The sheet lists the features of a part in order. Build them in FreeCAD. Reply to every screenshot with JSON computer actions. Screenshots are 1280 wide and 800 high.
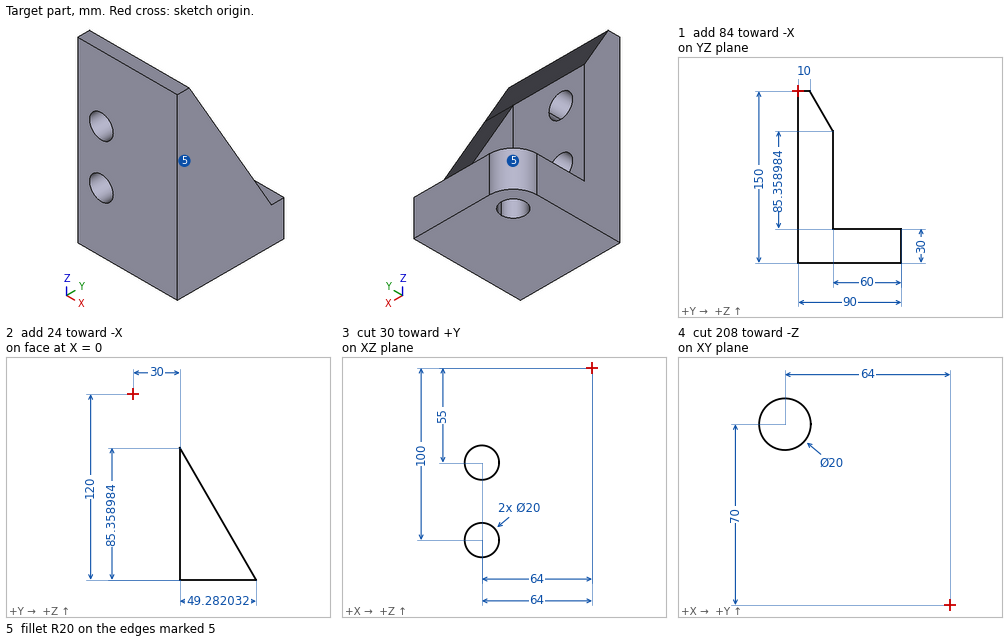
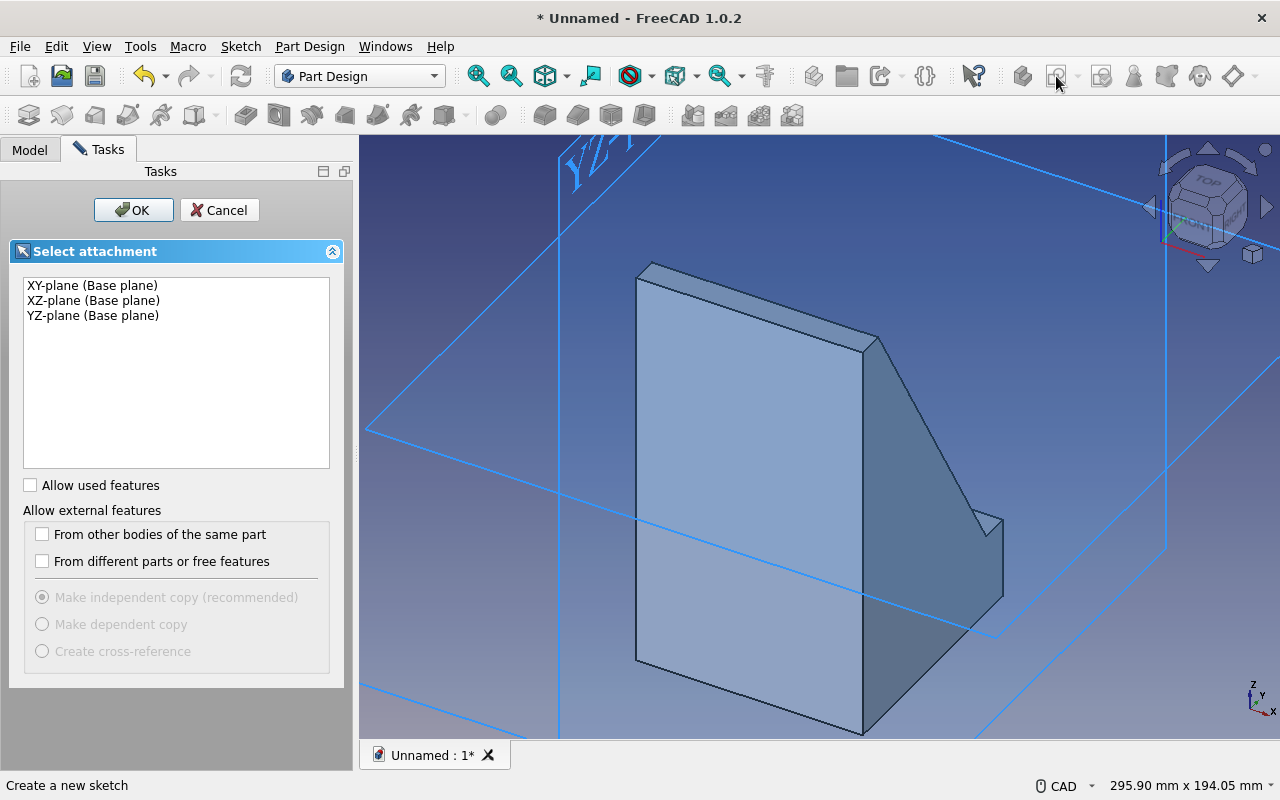
{"action": "left_click", "coordinate": [84, 300]}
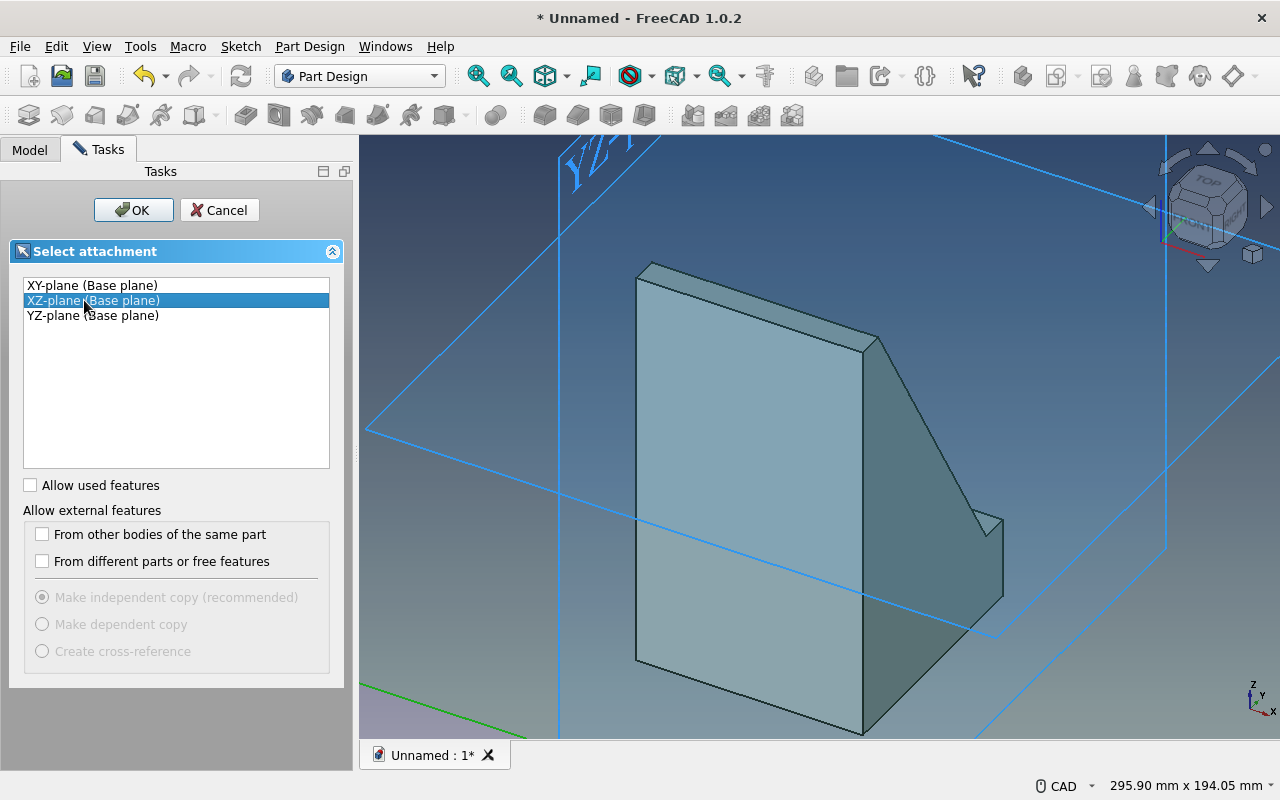
{"action": "left_click", "coordinate": [134, 210]}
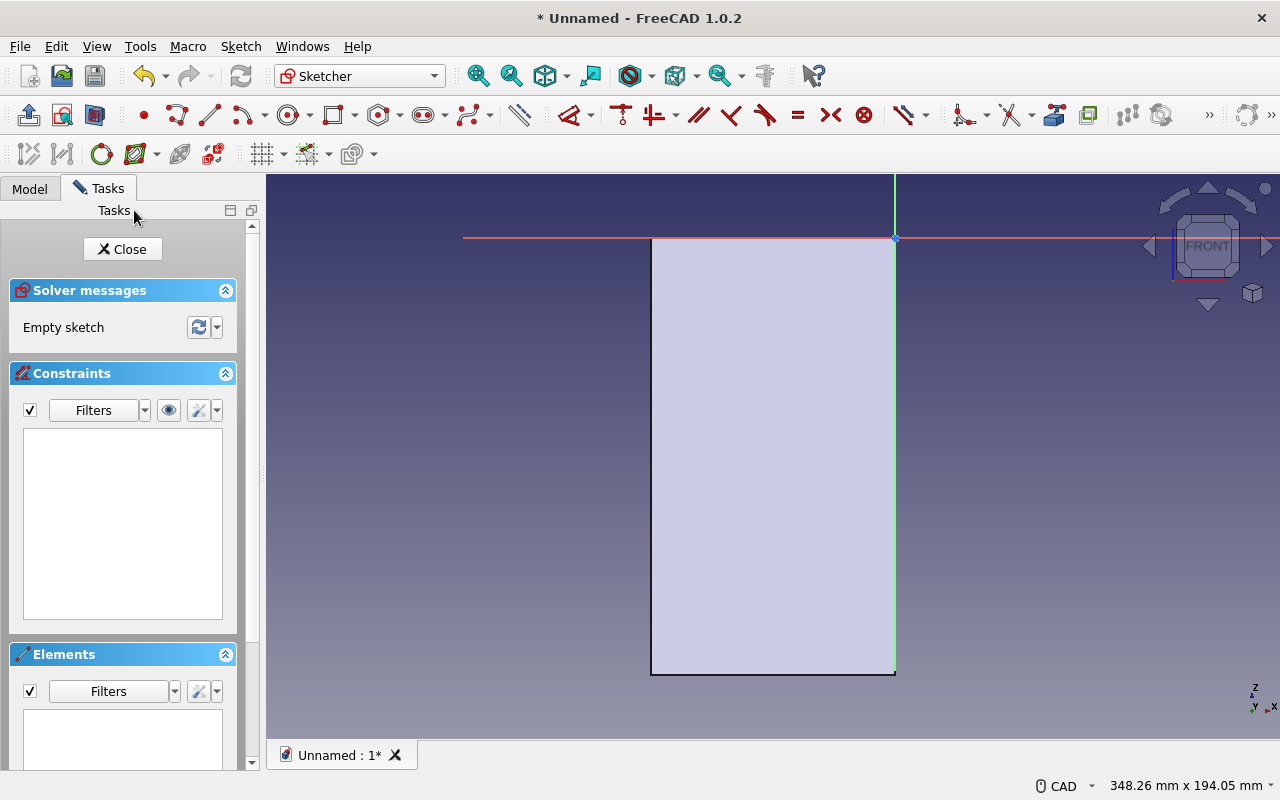
{"action": "left_click", "coordinate": [288, 116]}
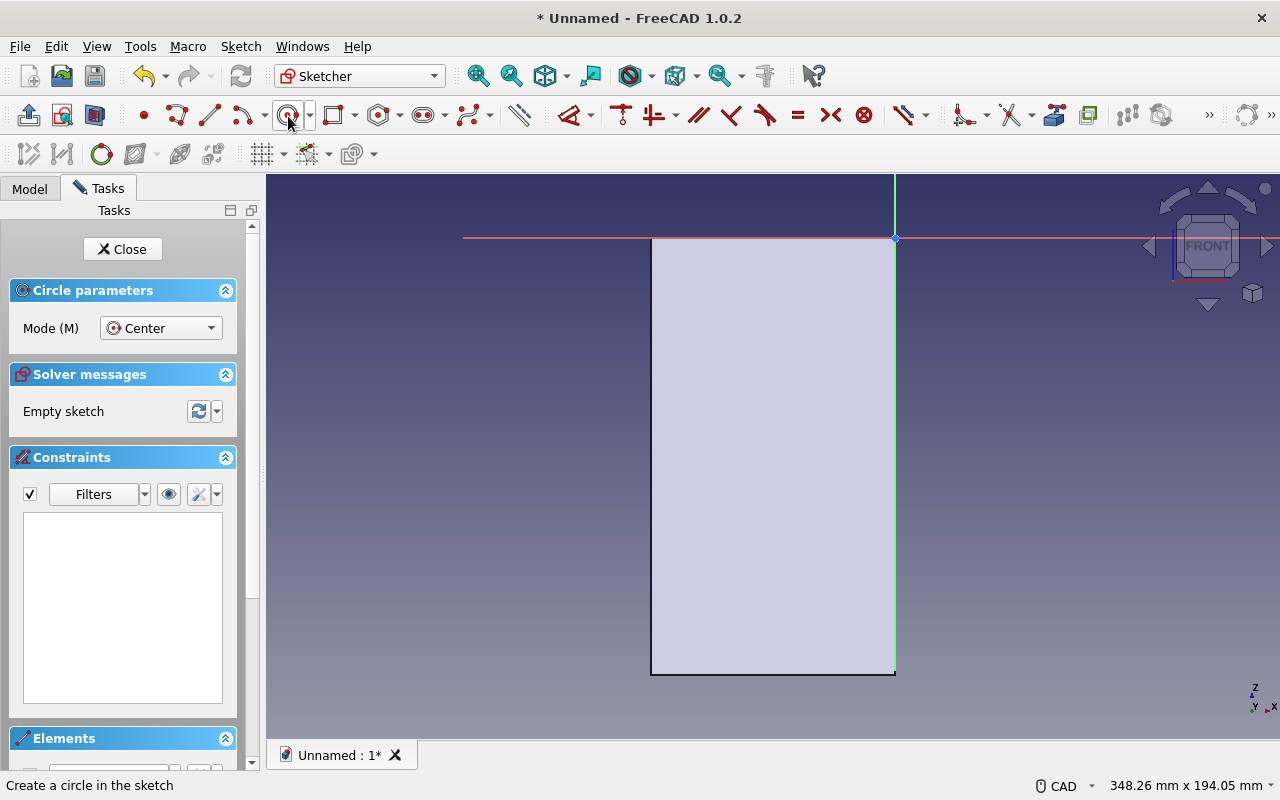
{"action": "left_click", "coordinate": [709, 529]}
{"action": "left_click", "coordinate": [730, 509]}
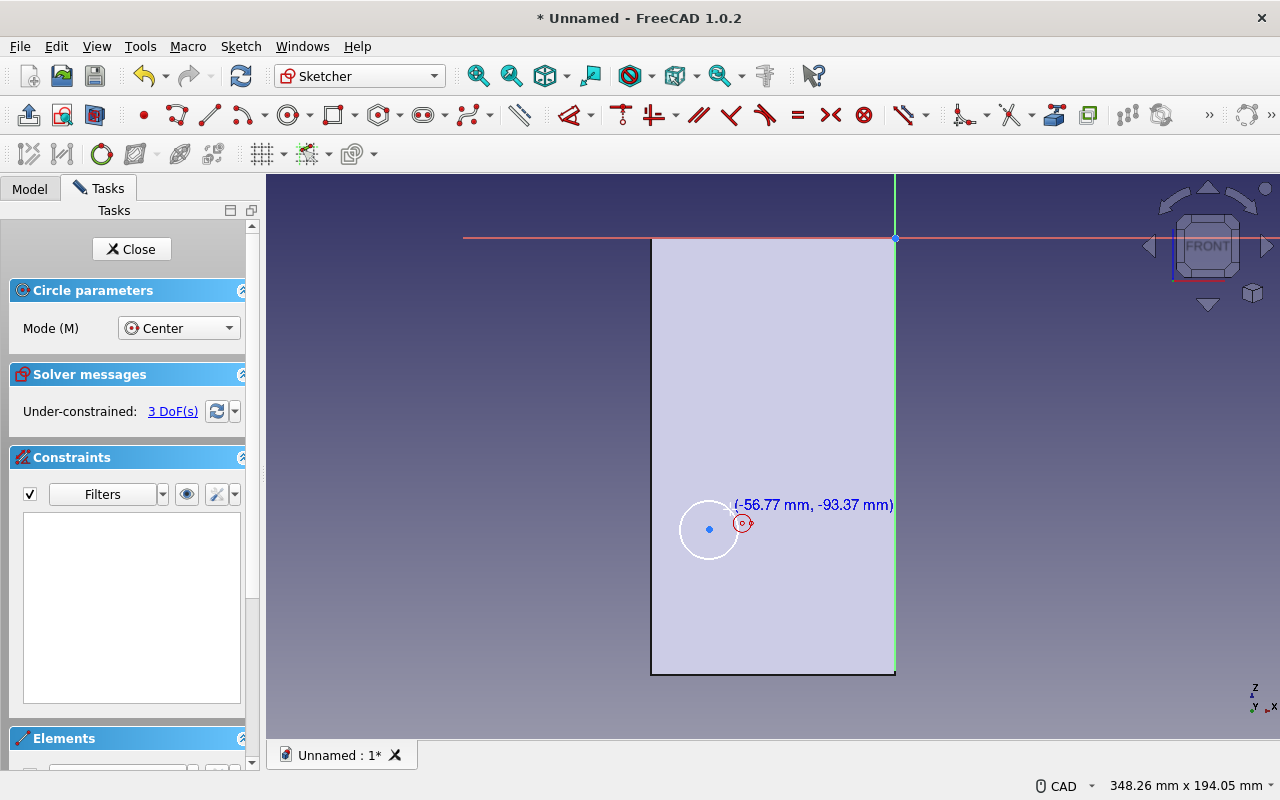
{"action": "left_click", "coordinate": [709, 398]}
{"action": "left_click", "coordinate": [730, 378]}
{"action": "key", "text": "Escape"}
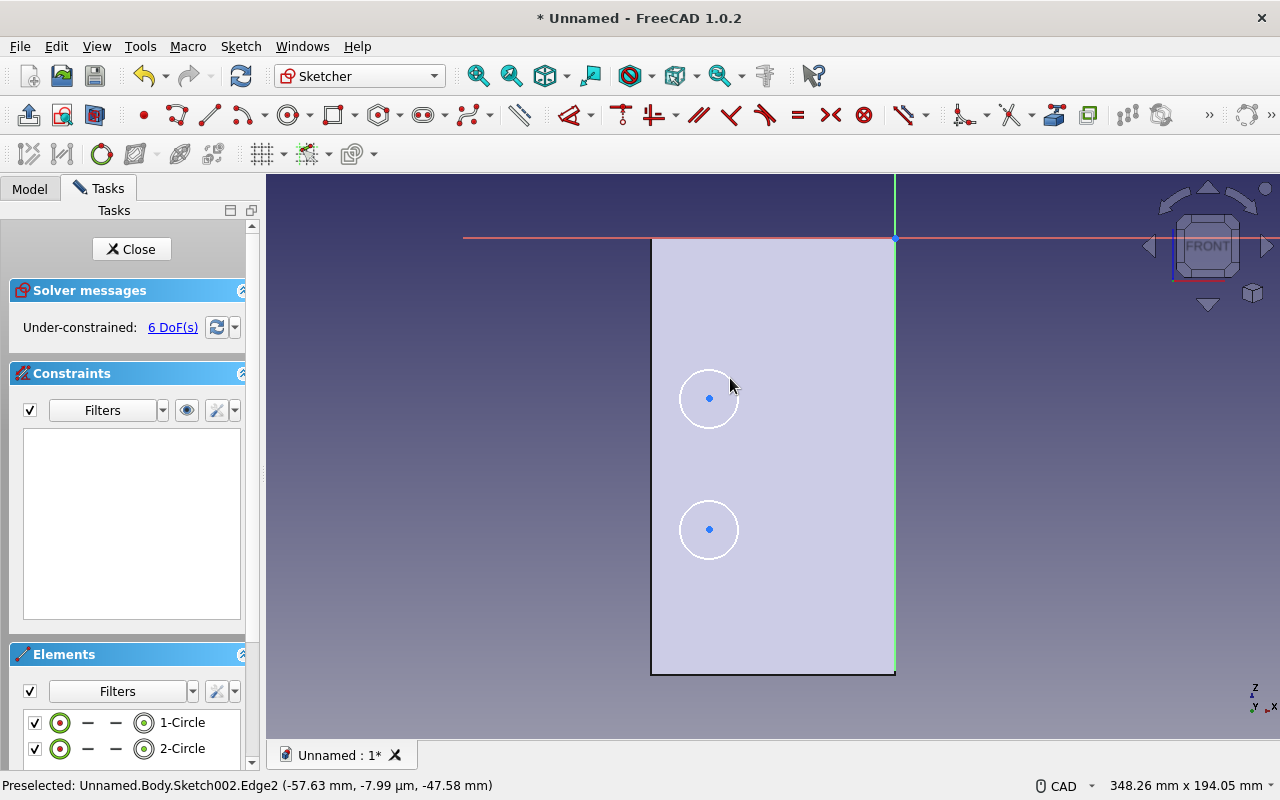
{"action": "left_click", "coordinate": [729, 509]}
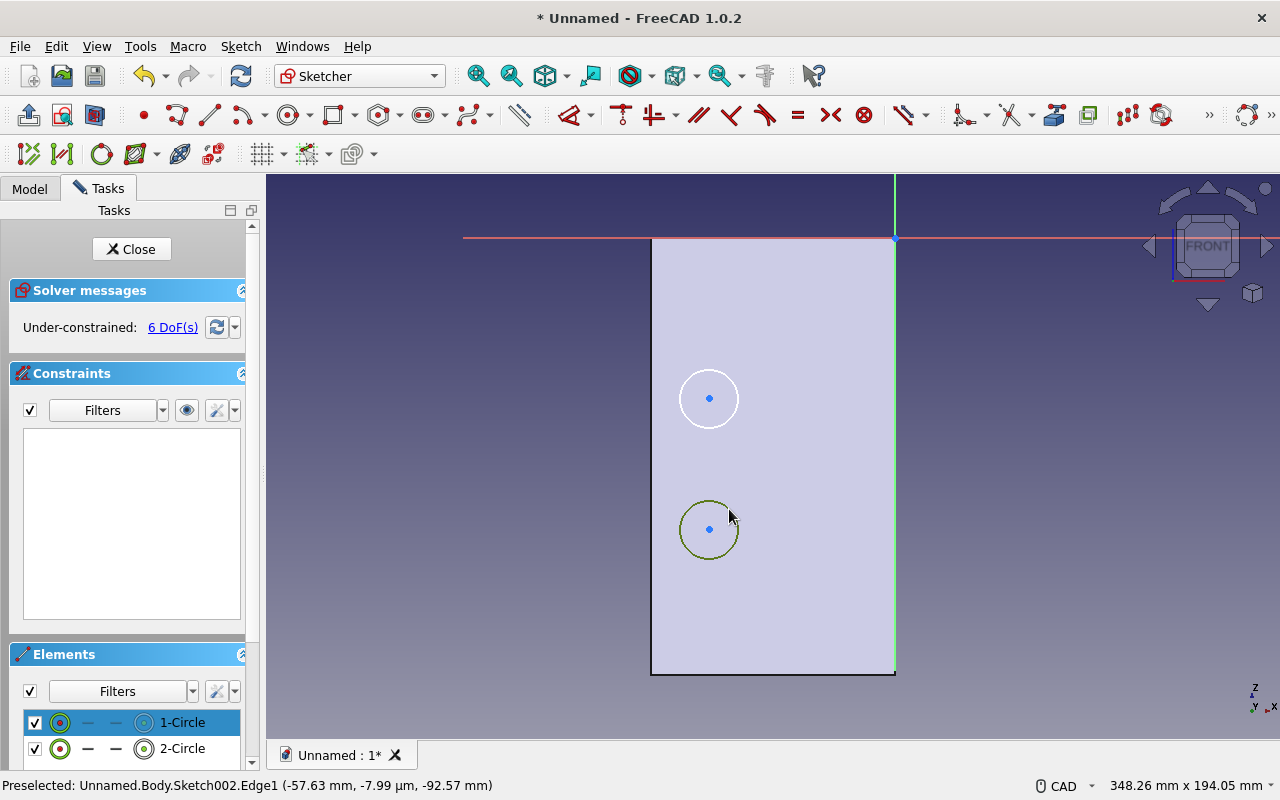
{"action": "left_click", "coordinate": [729, 378]}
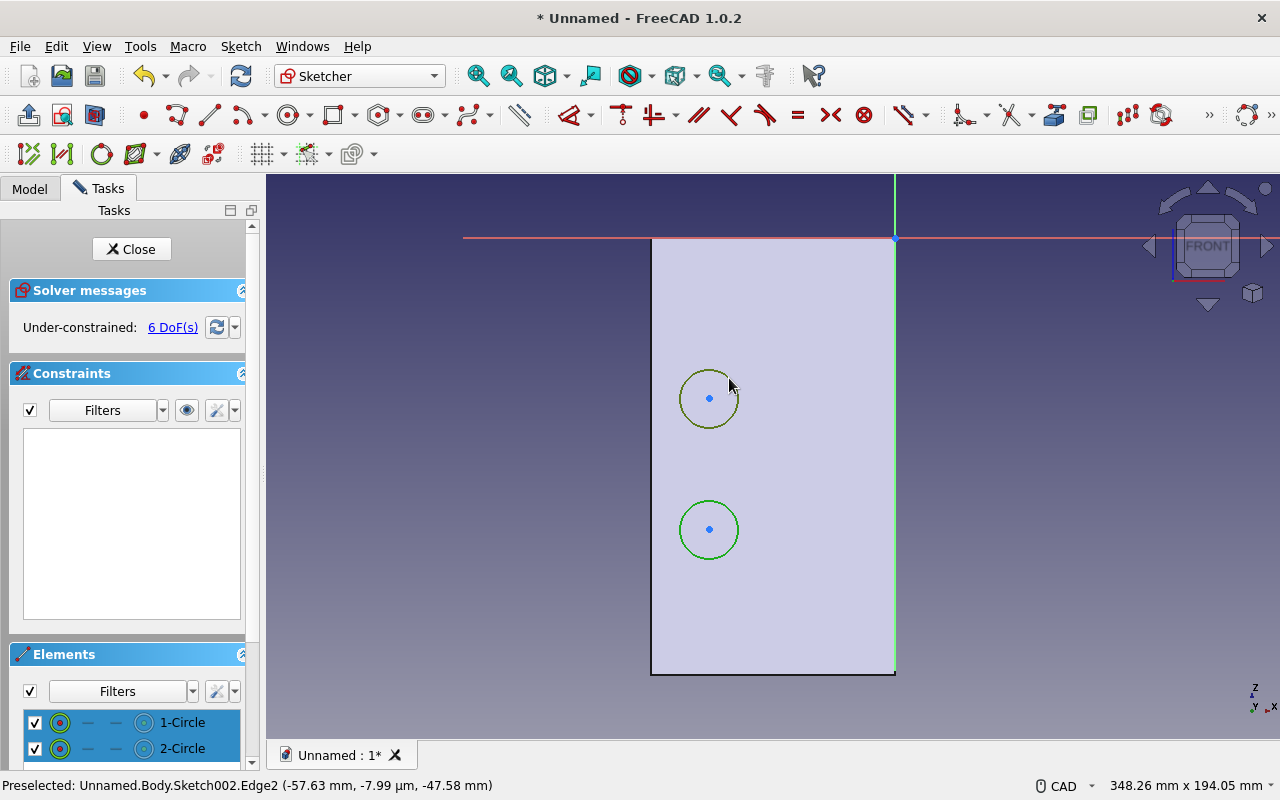
{"action": "left_click", "coordinate": [798, 116]}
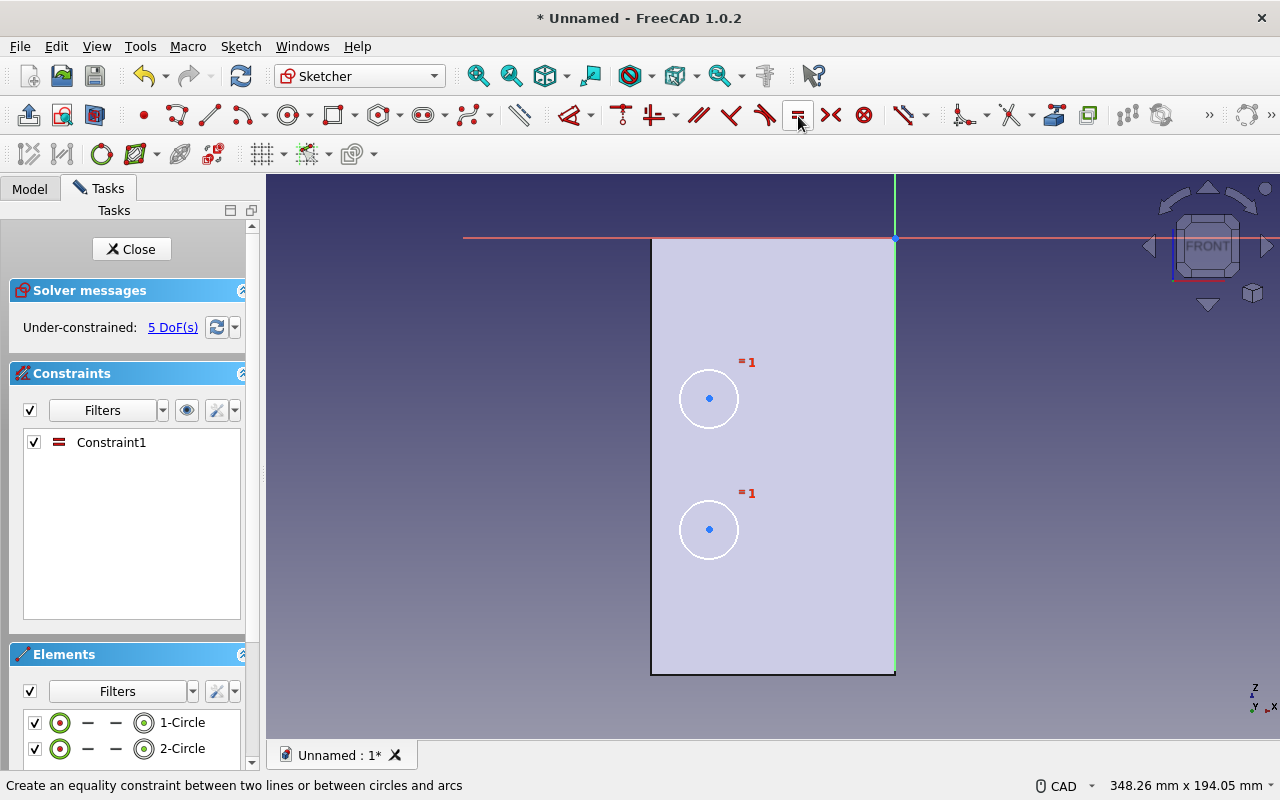
{"action": "left_click", "coordinate": [568, 116]}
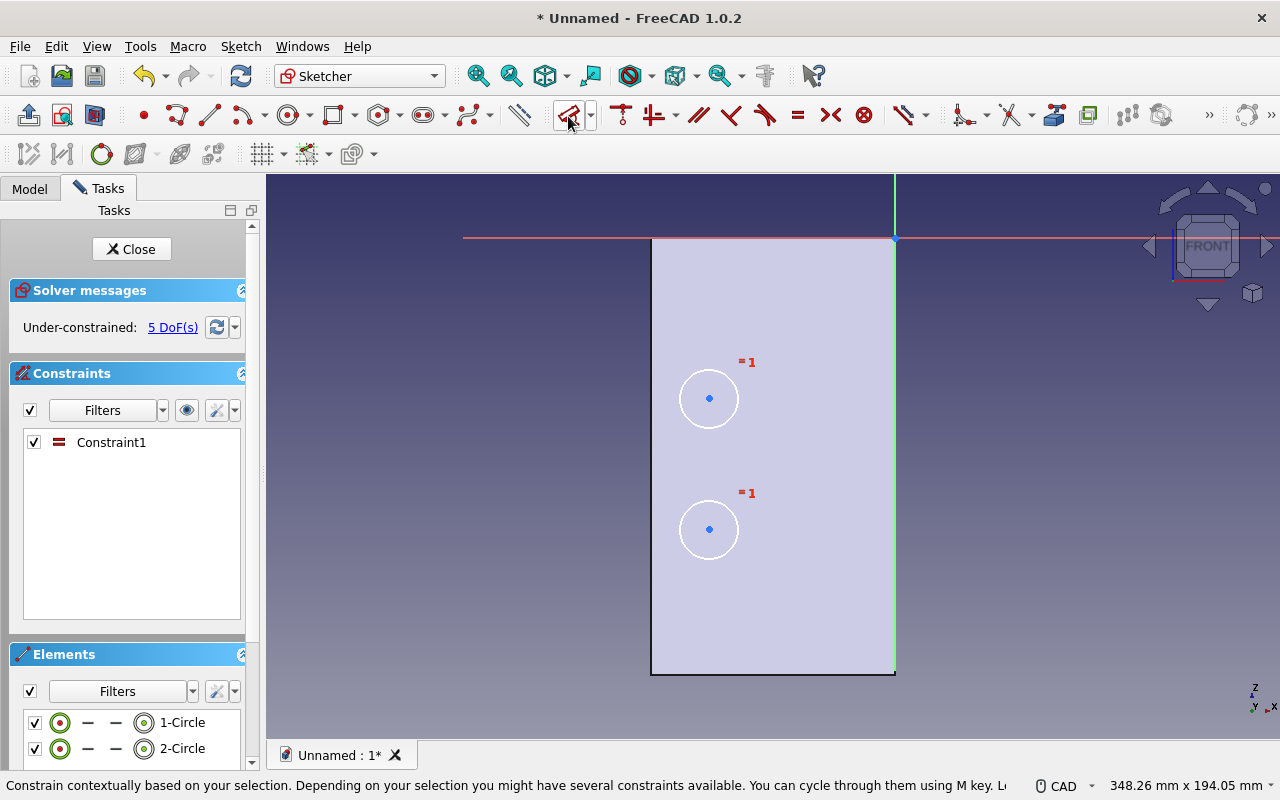
{"action": "left_click", "coordinate": [729, 509]}
{"action": "left_click", "coordinate": [751, 486]}